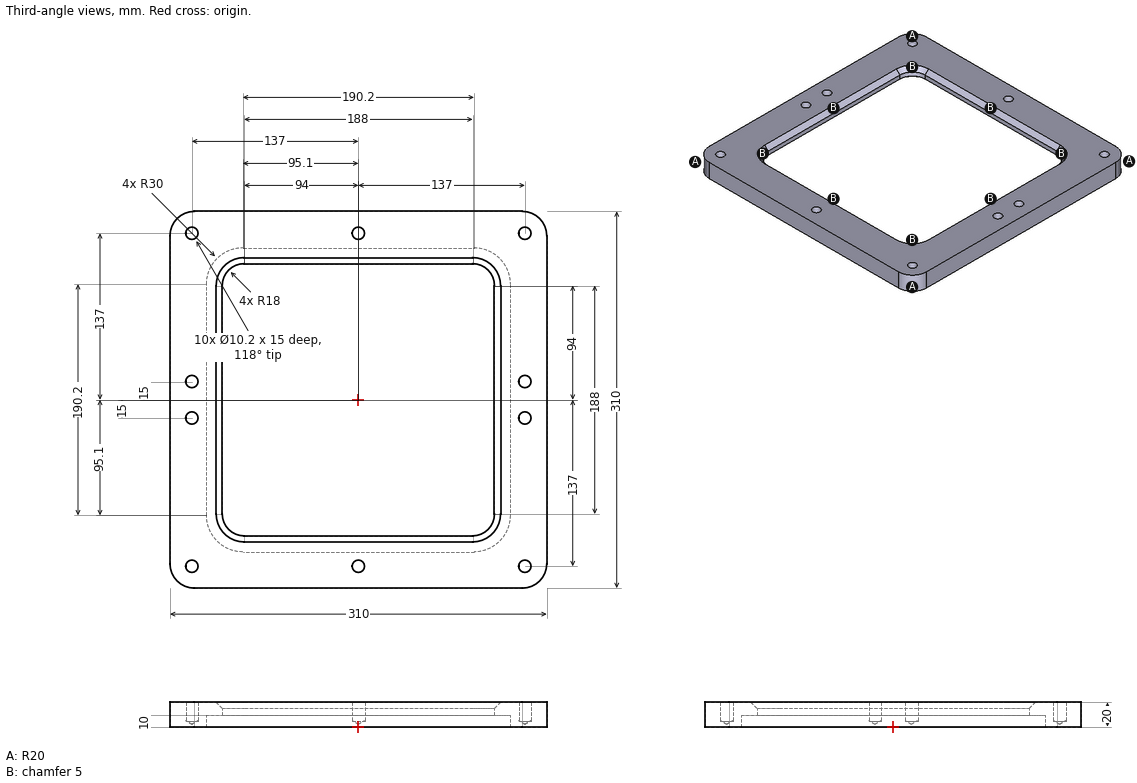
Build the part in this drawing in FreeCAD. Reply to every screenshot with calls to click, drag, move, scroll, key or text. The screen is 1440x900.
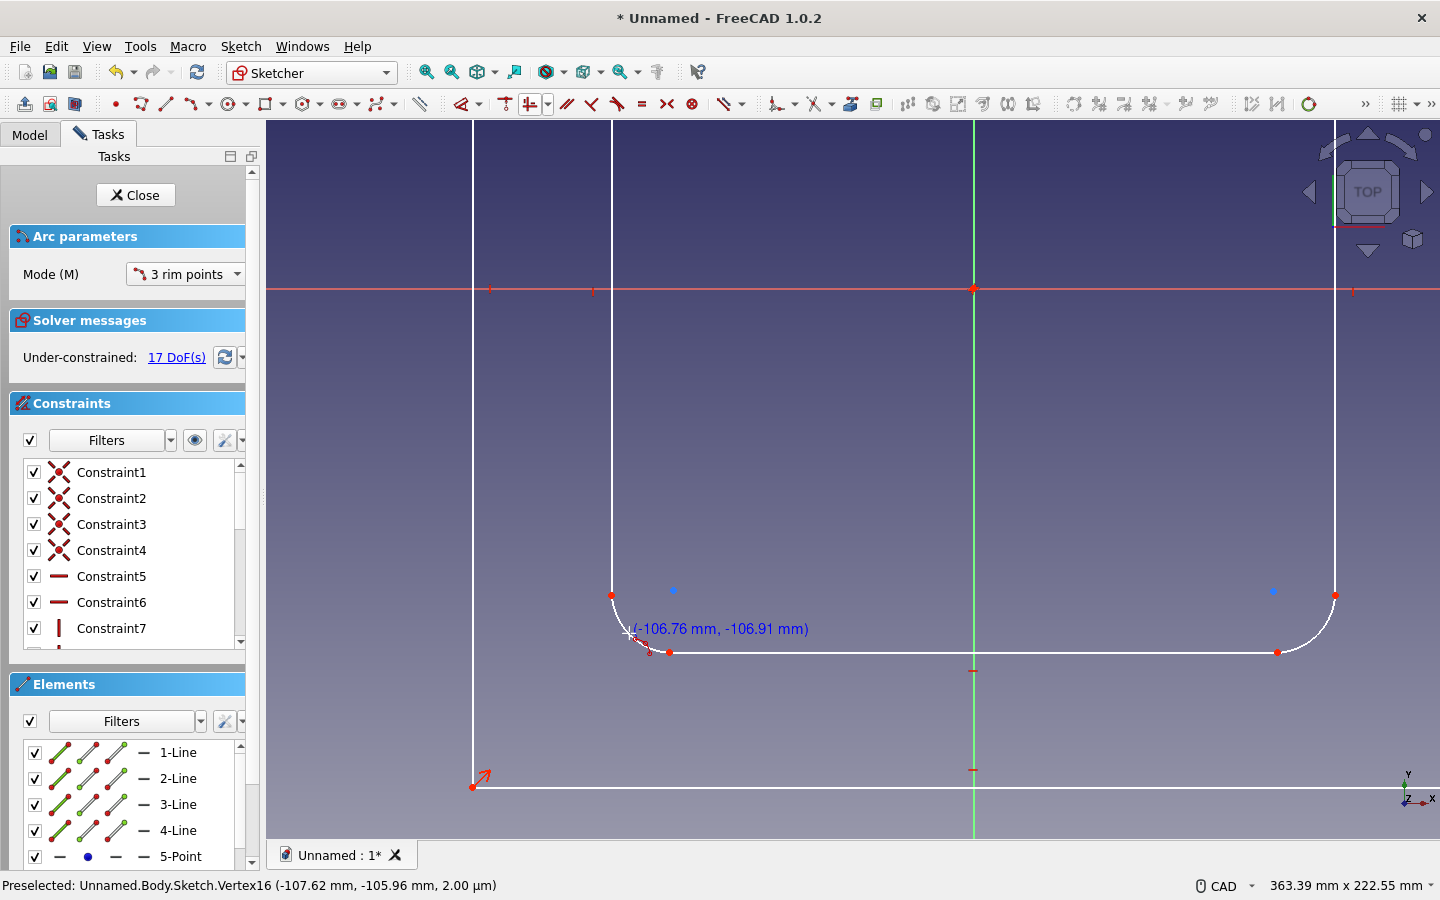
scroll(630, 635, down, 4)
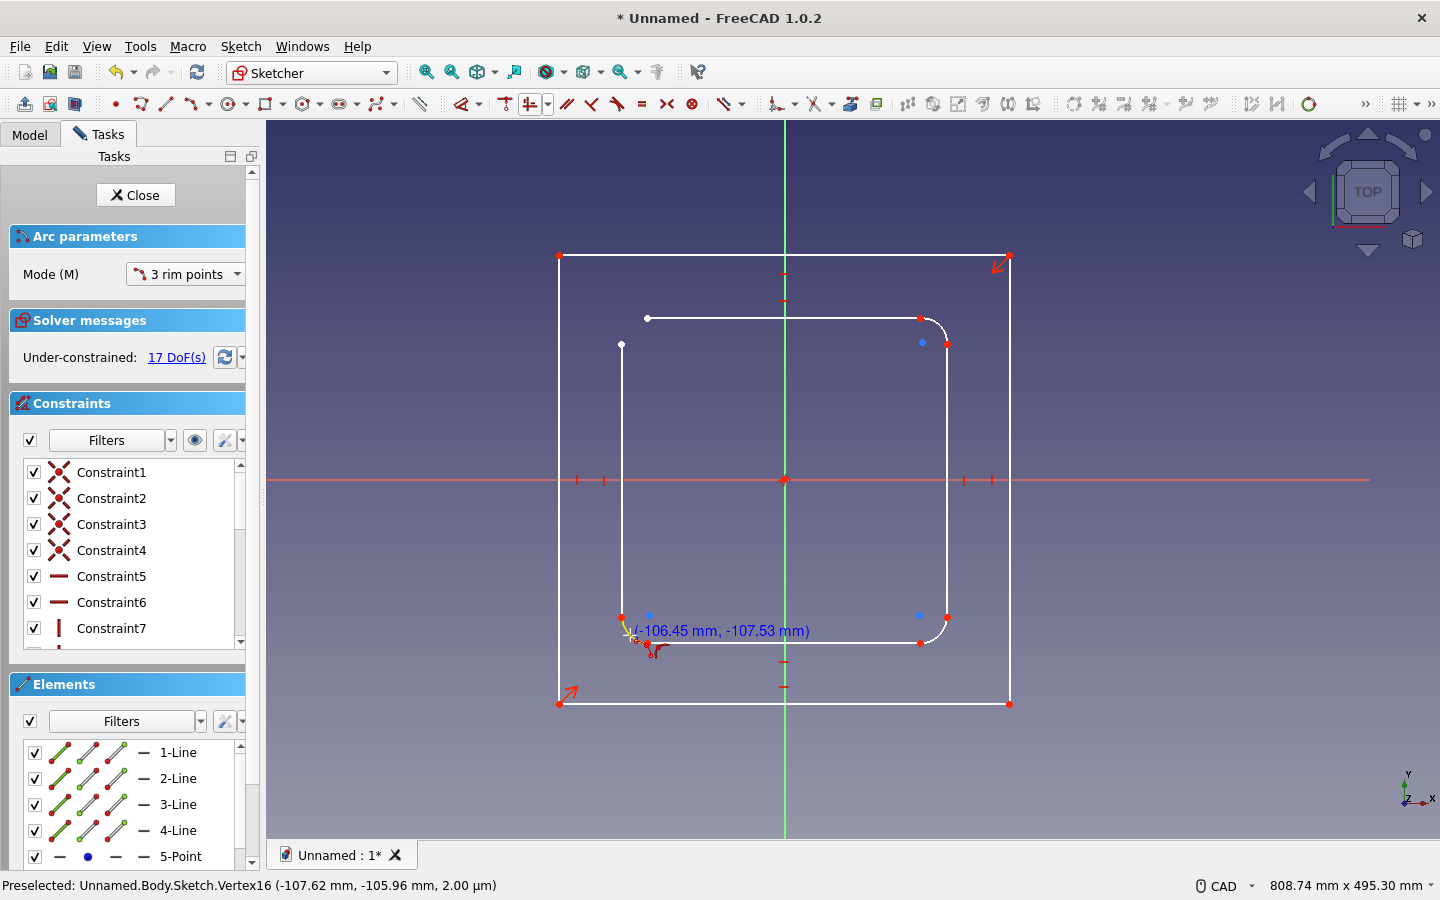
click(622, 344)
click(648, 318)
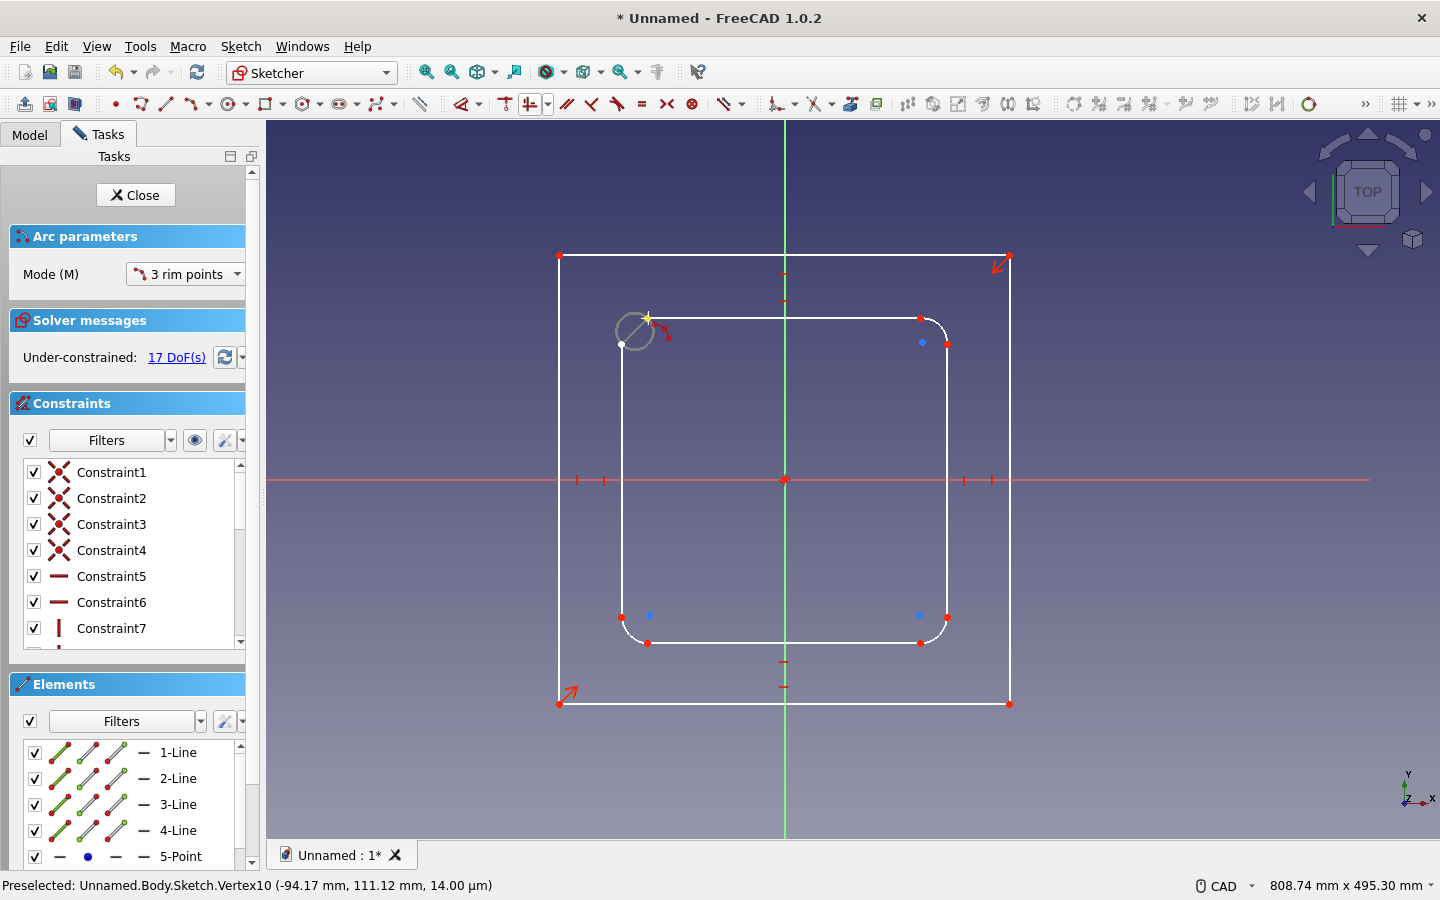
scroll(630, 325, up, 4)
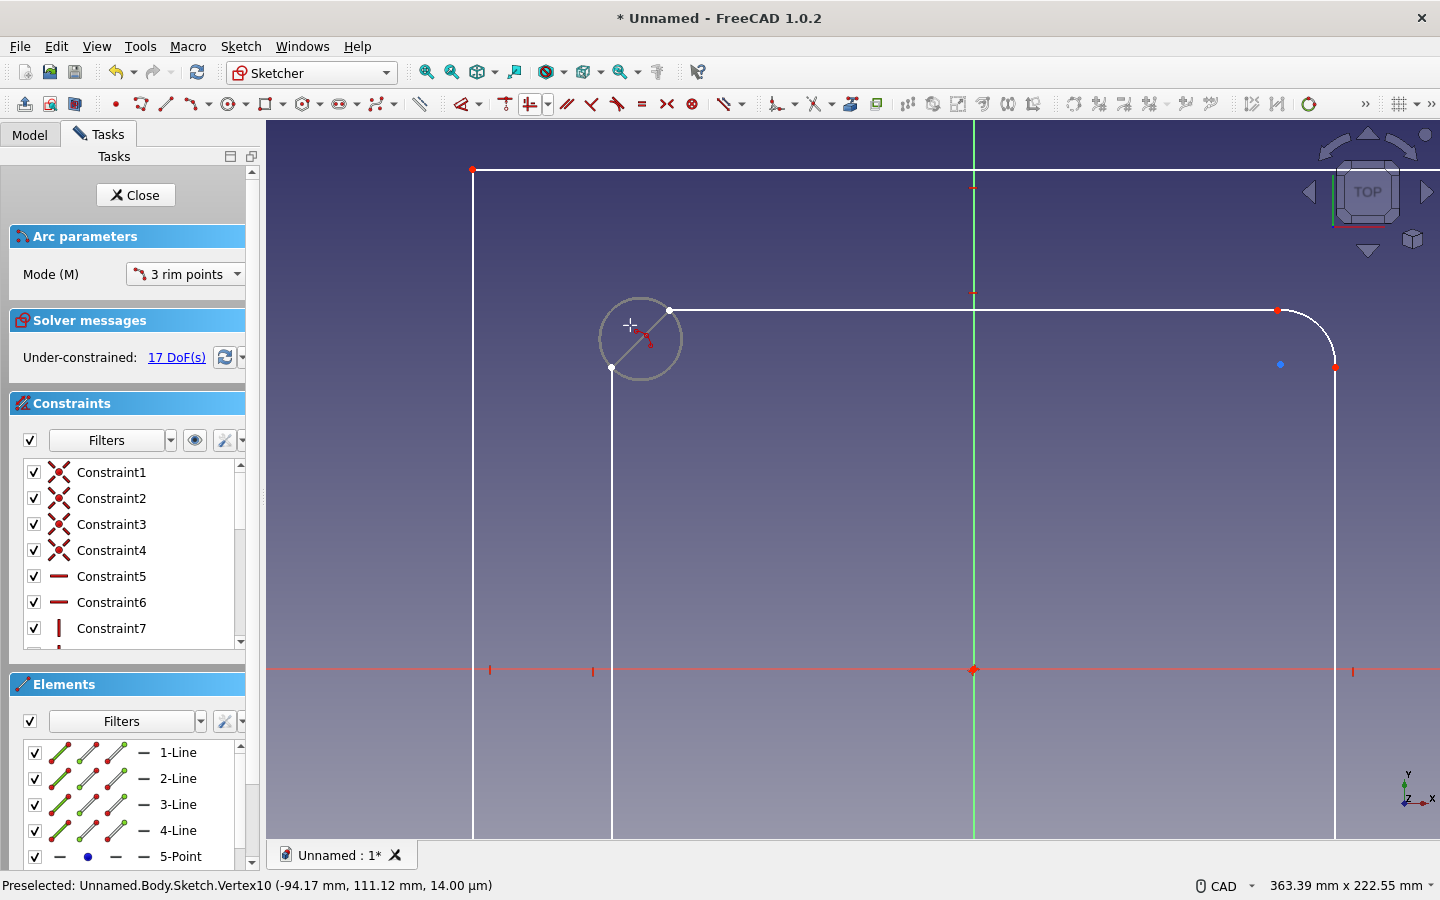
click(629, 324)
key(Escape)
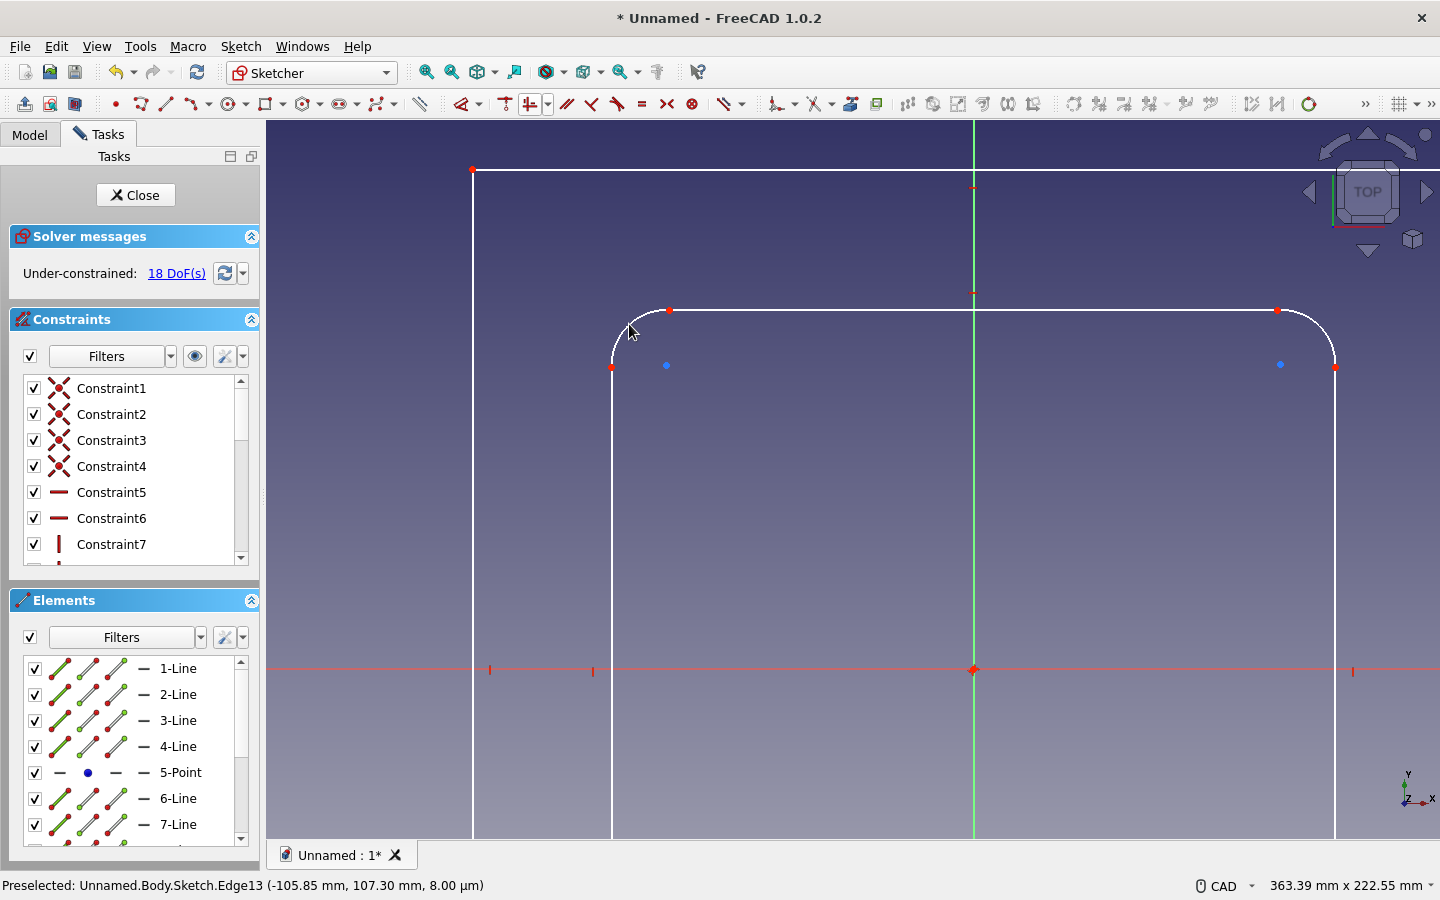
click(852, 310)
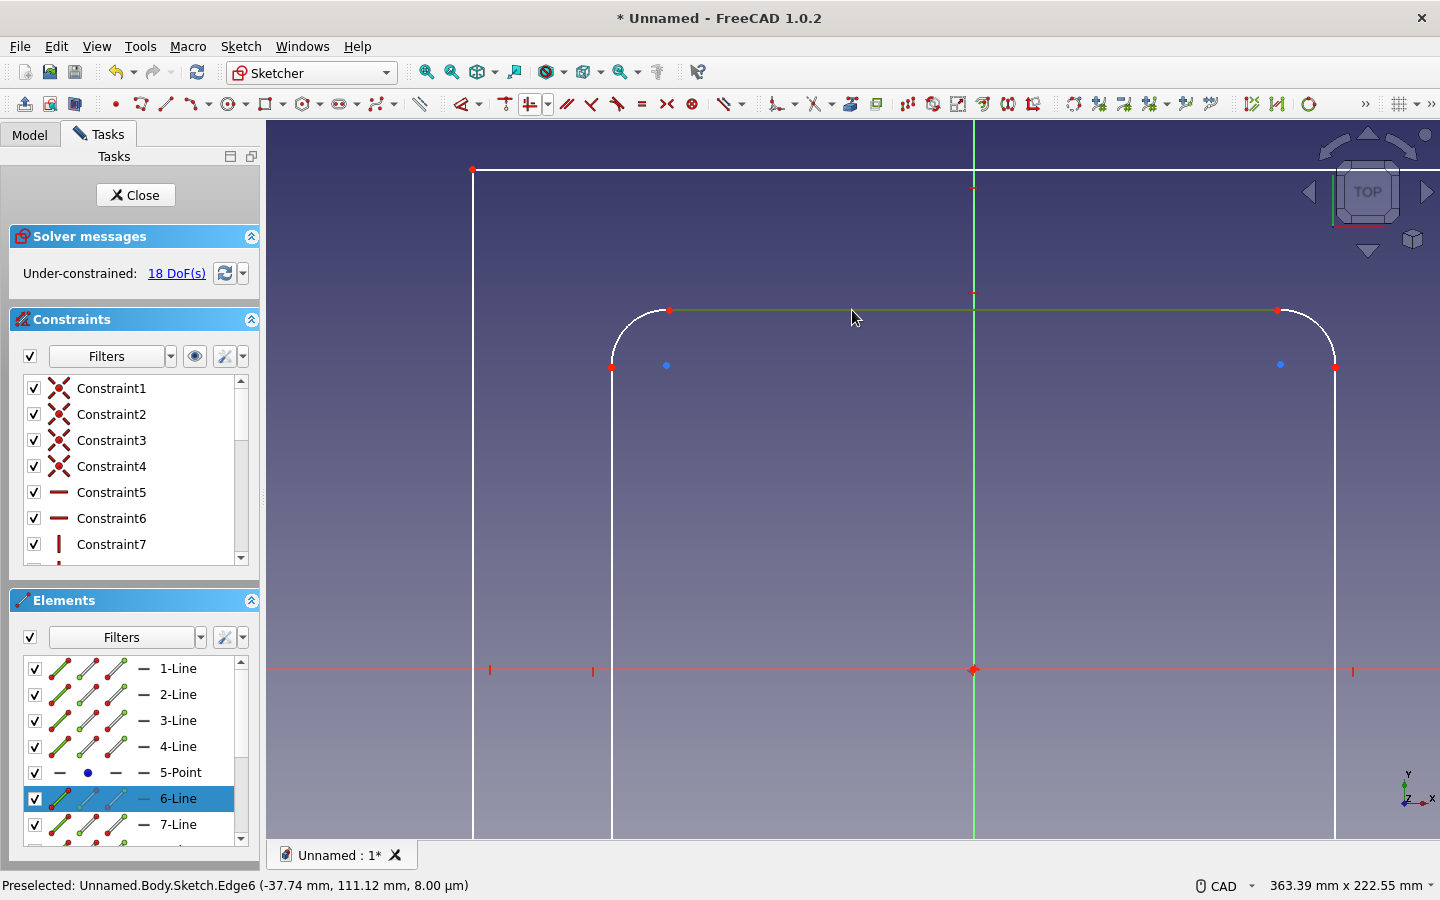
scroll(630, 325, down, 4)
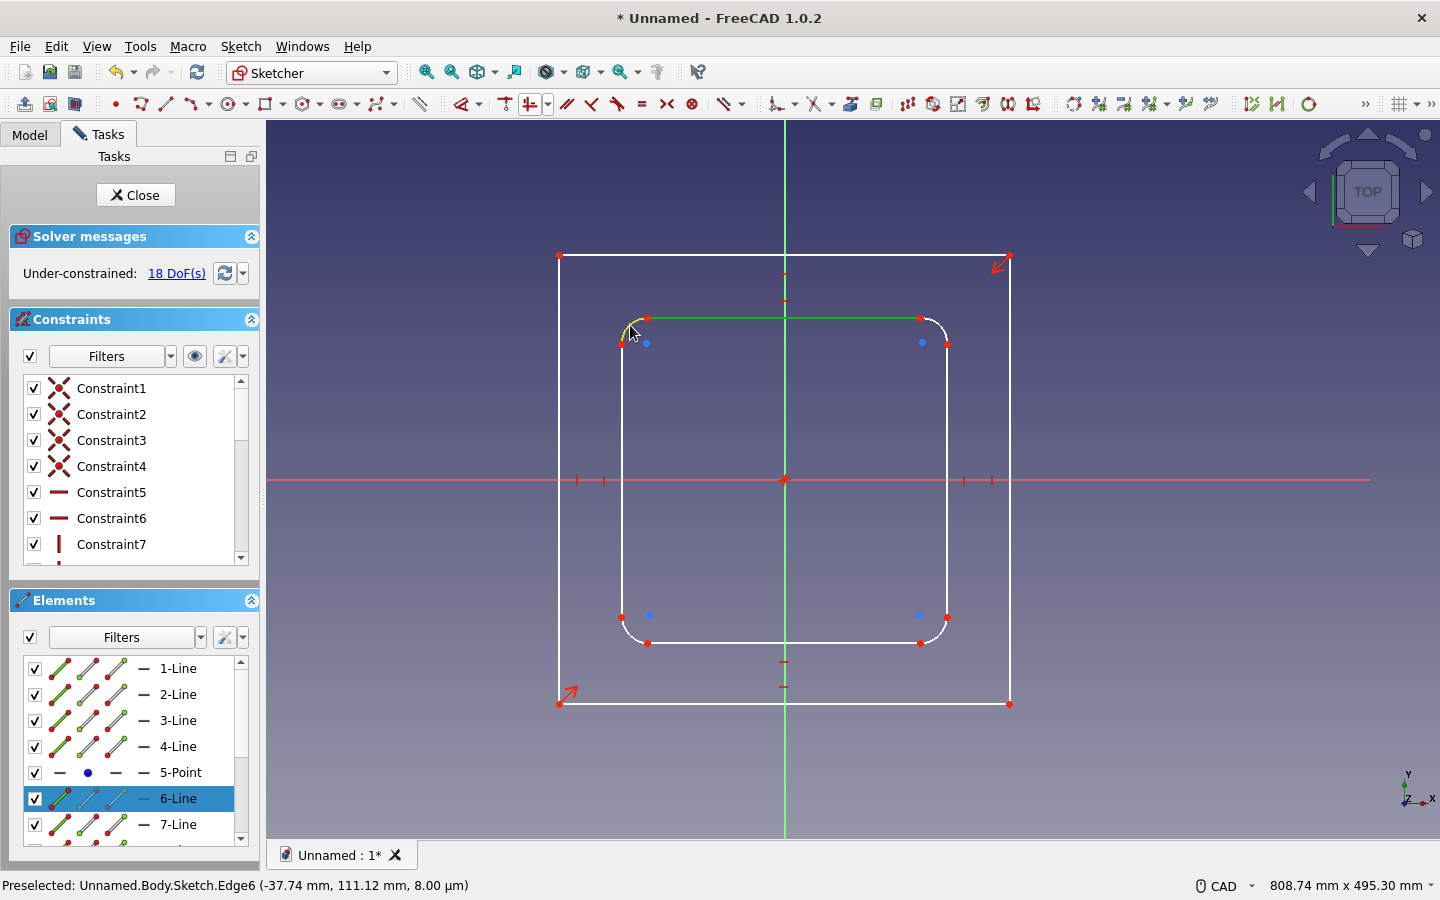
click(945, 332)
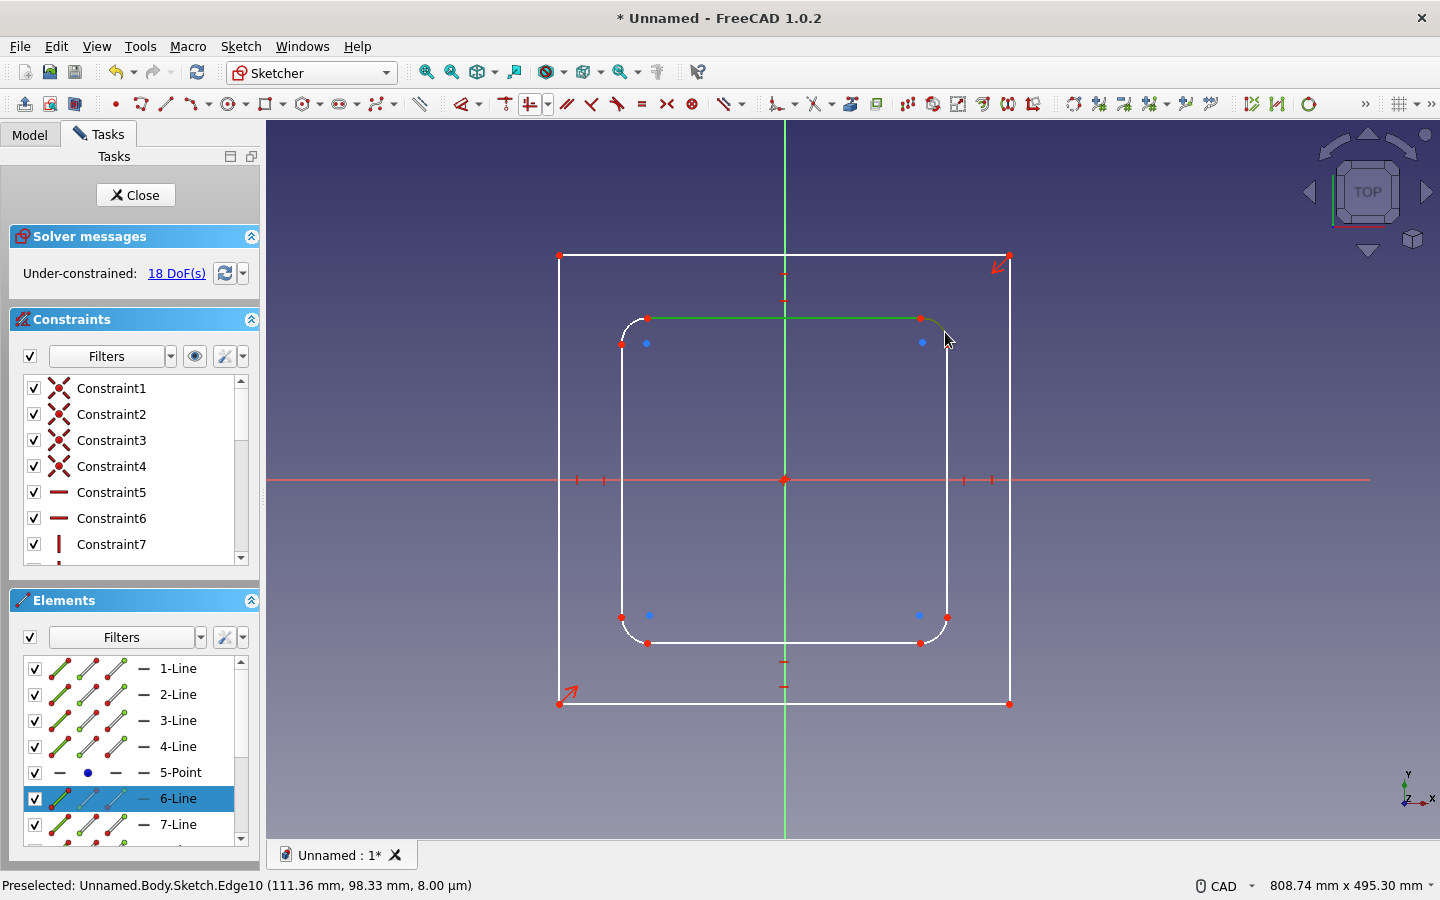
click(617, 104)